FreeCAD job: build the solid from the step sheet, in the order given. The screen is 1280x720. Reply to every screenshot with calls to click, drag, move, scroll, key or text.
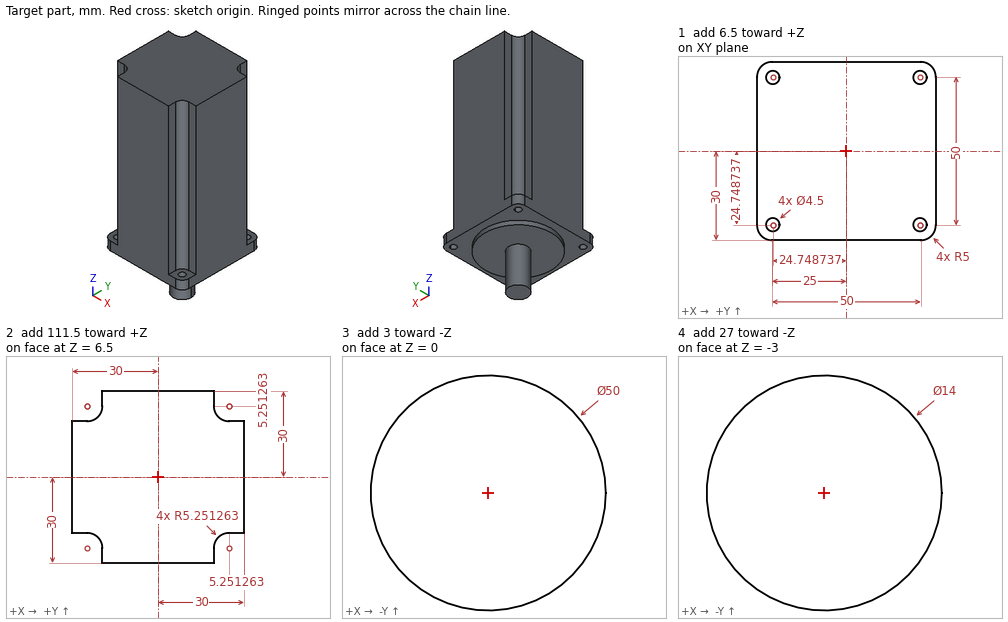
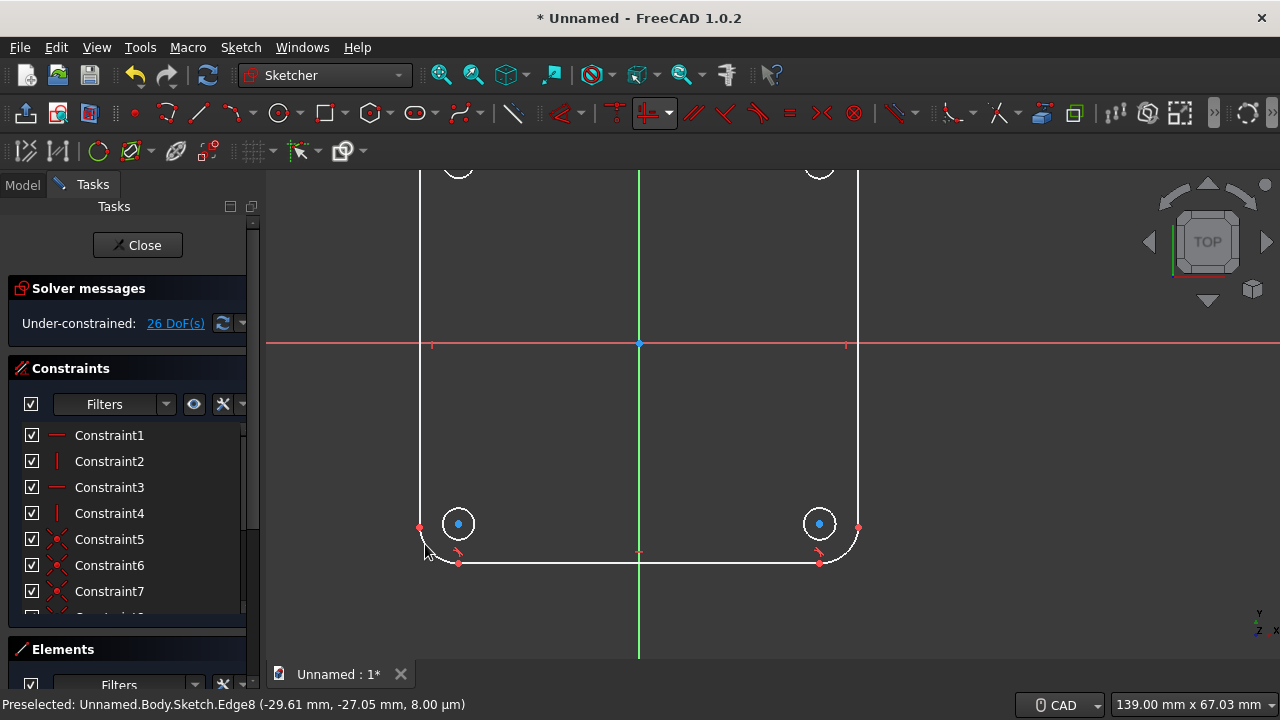
click(858, 418)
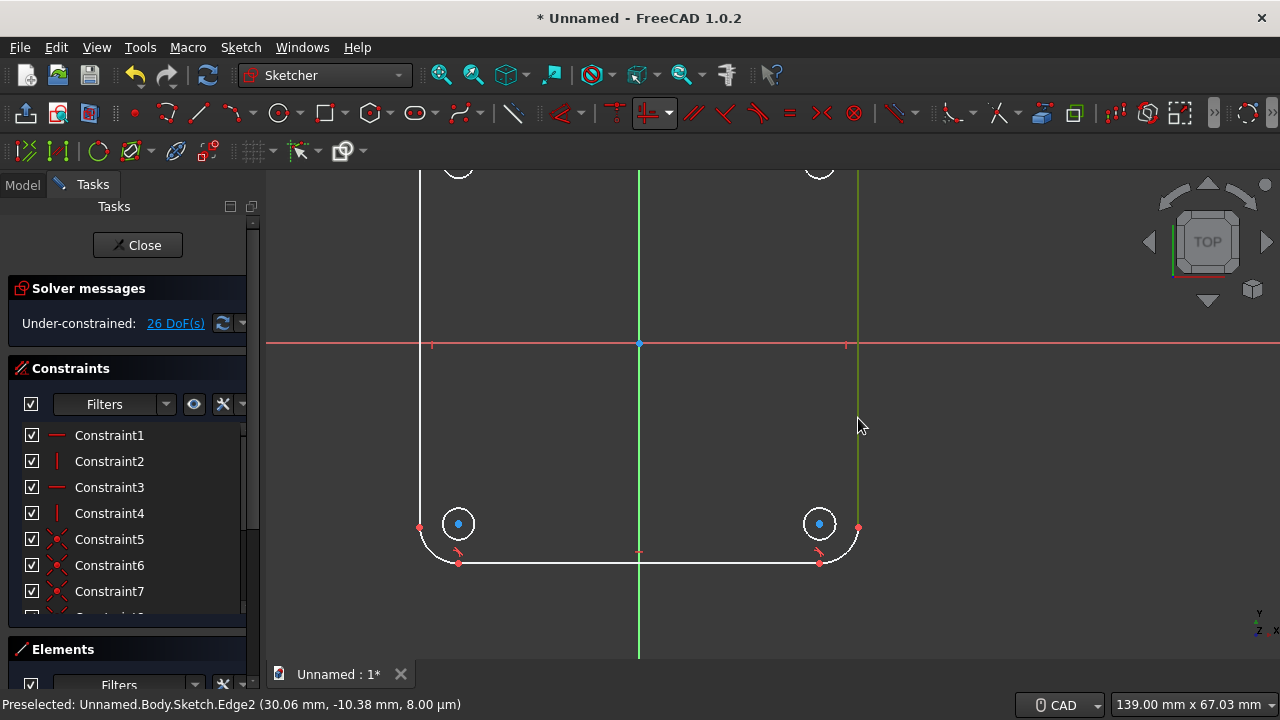
click(837, 560)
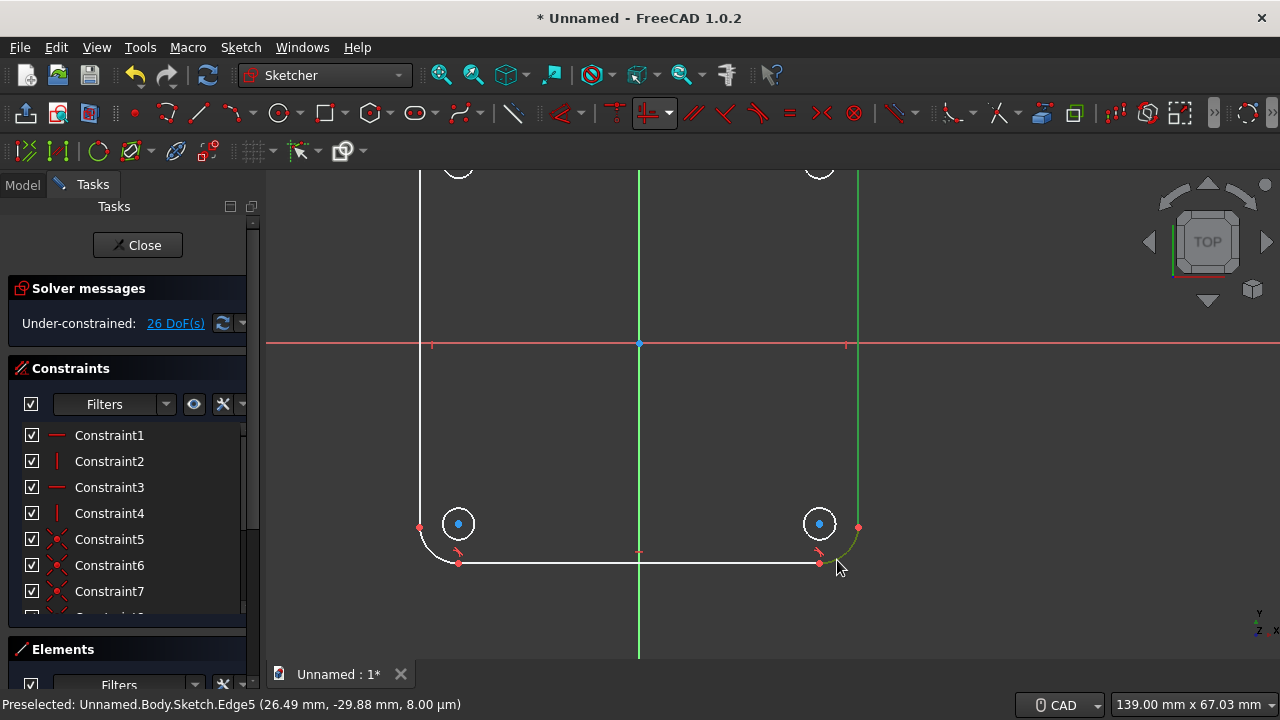
key(t)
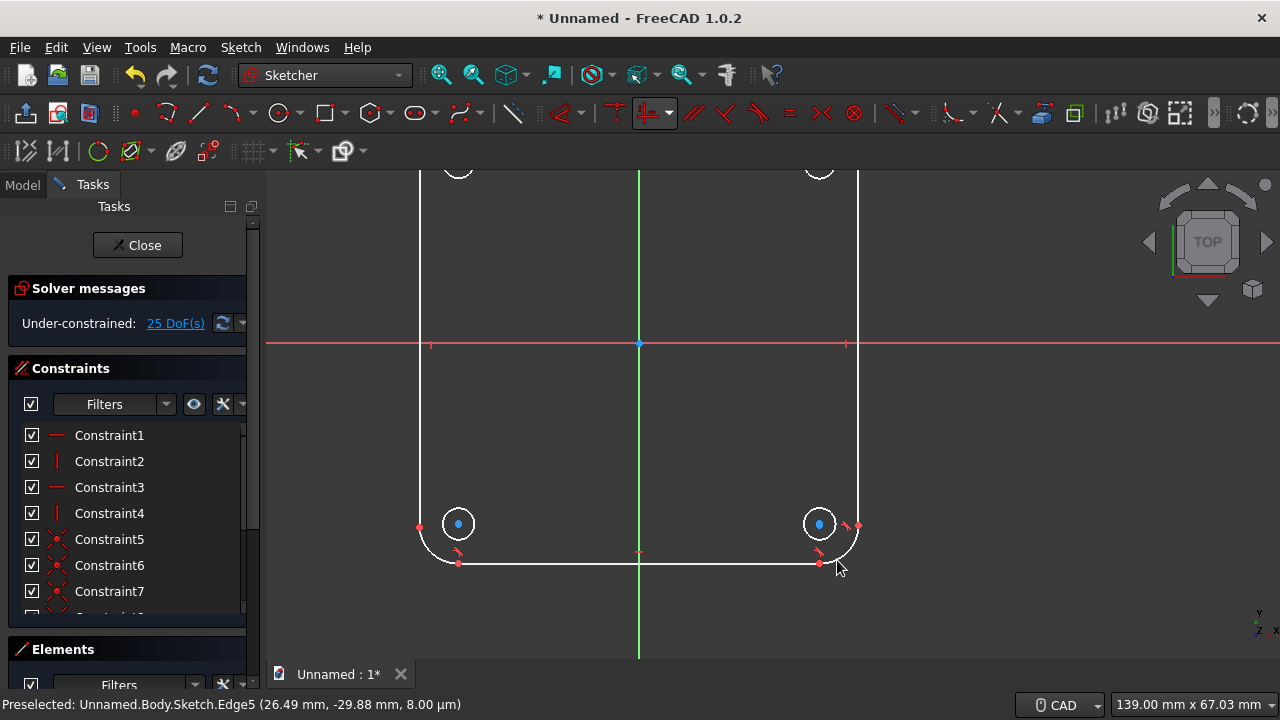
click(858, 416)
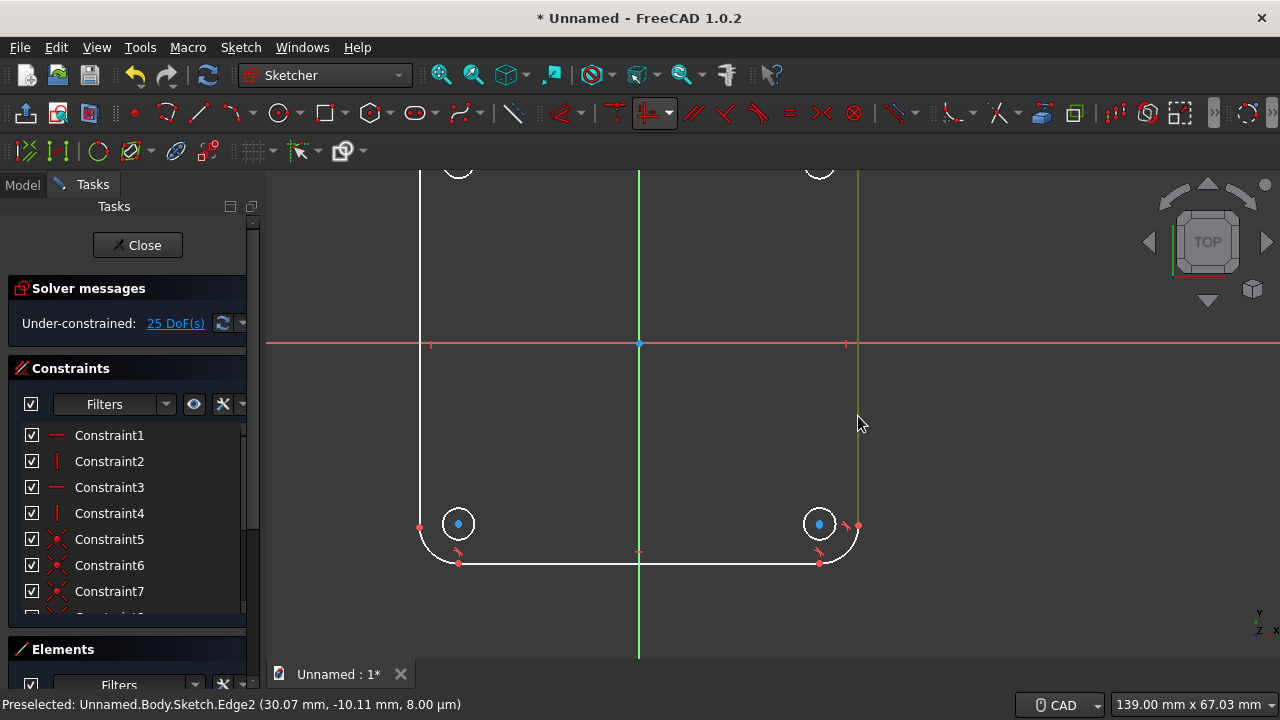
scroll(837, 559, down, 2)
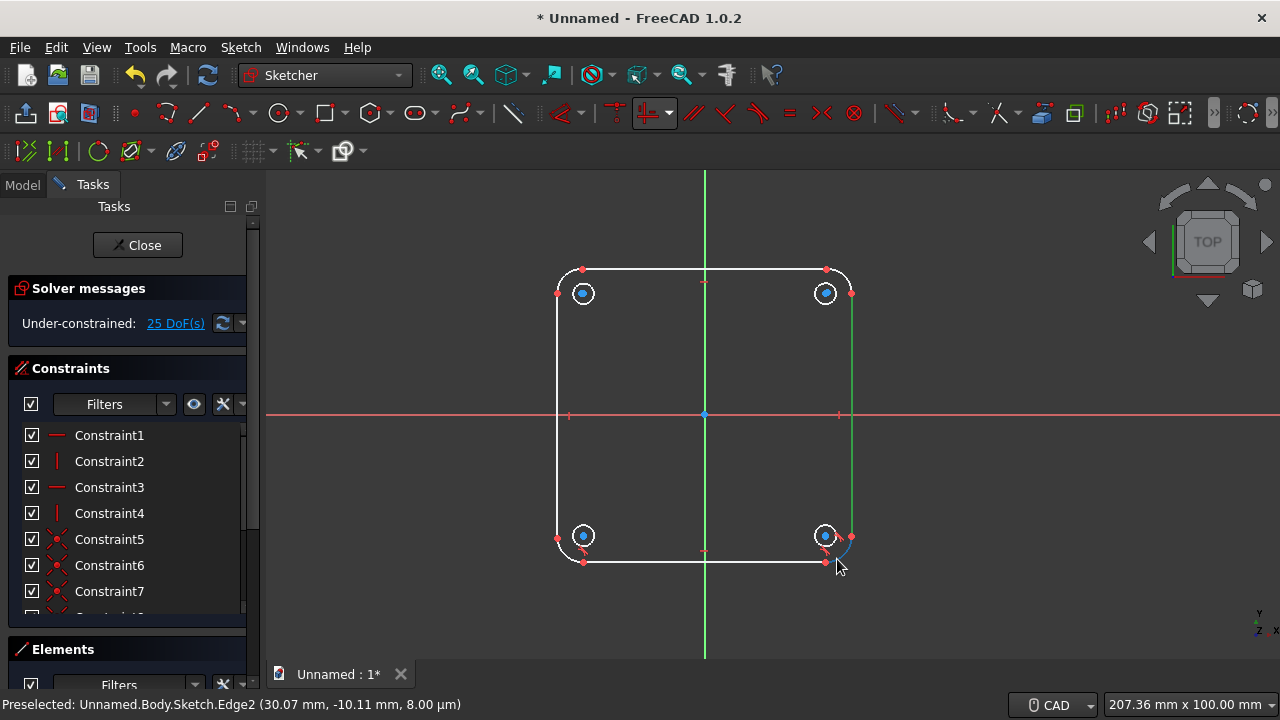
click(849, 282)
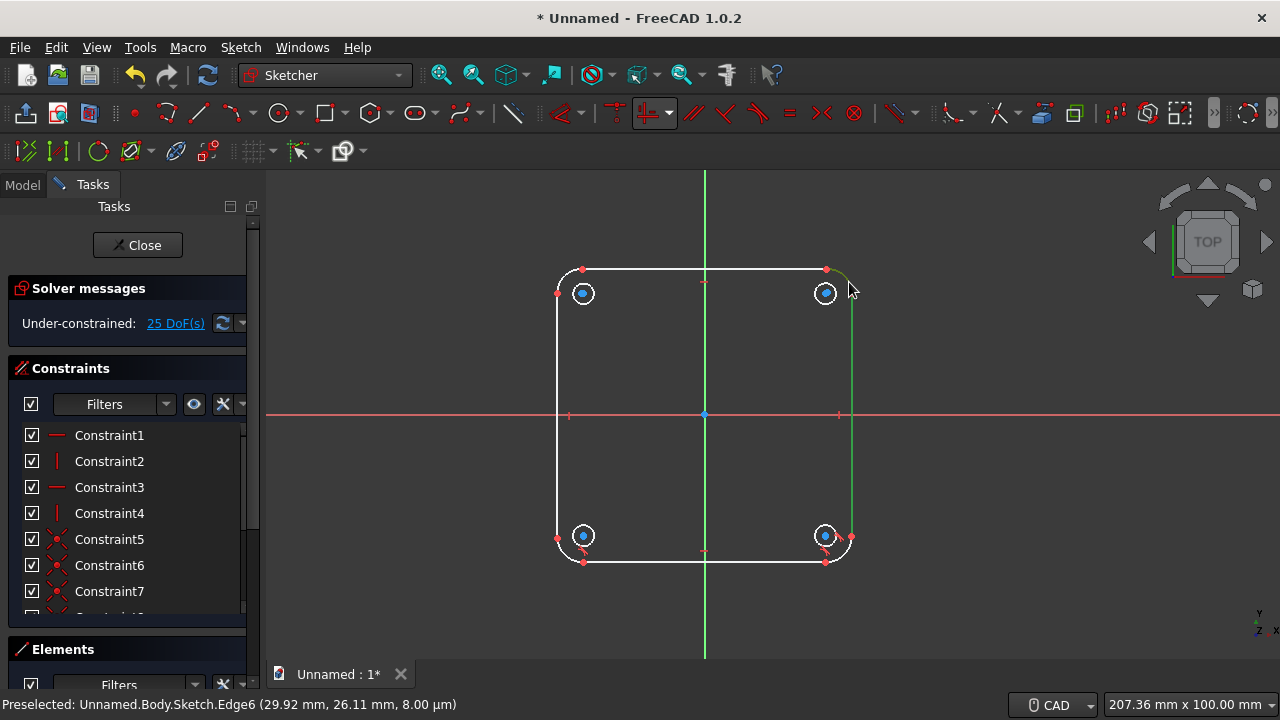
key(t)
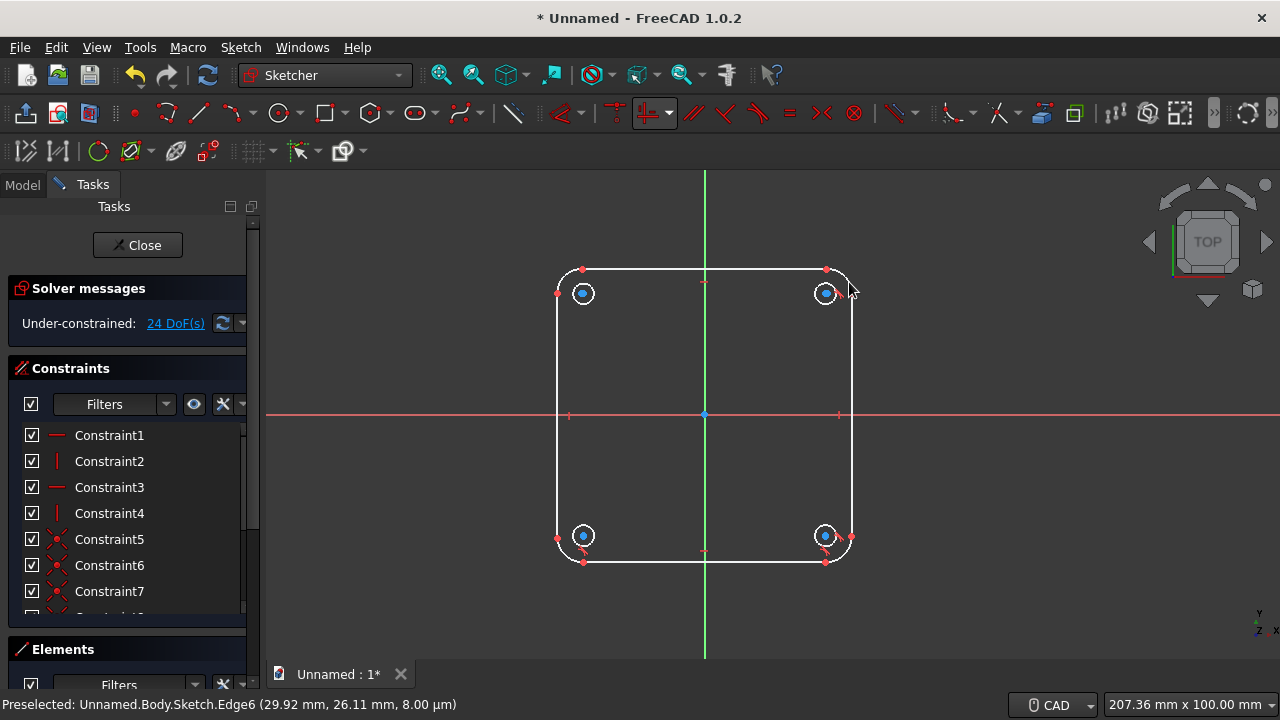
click(753, 269)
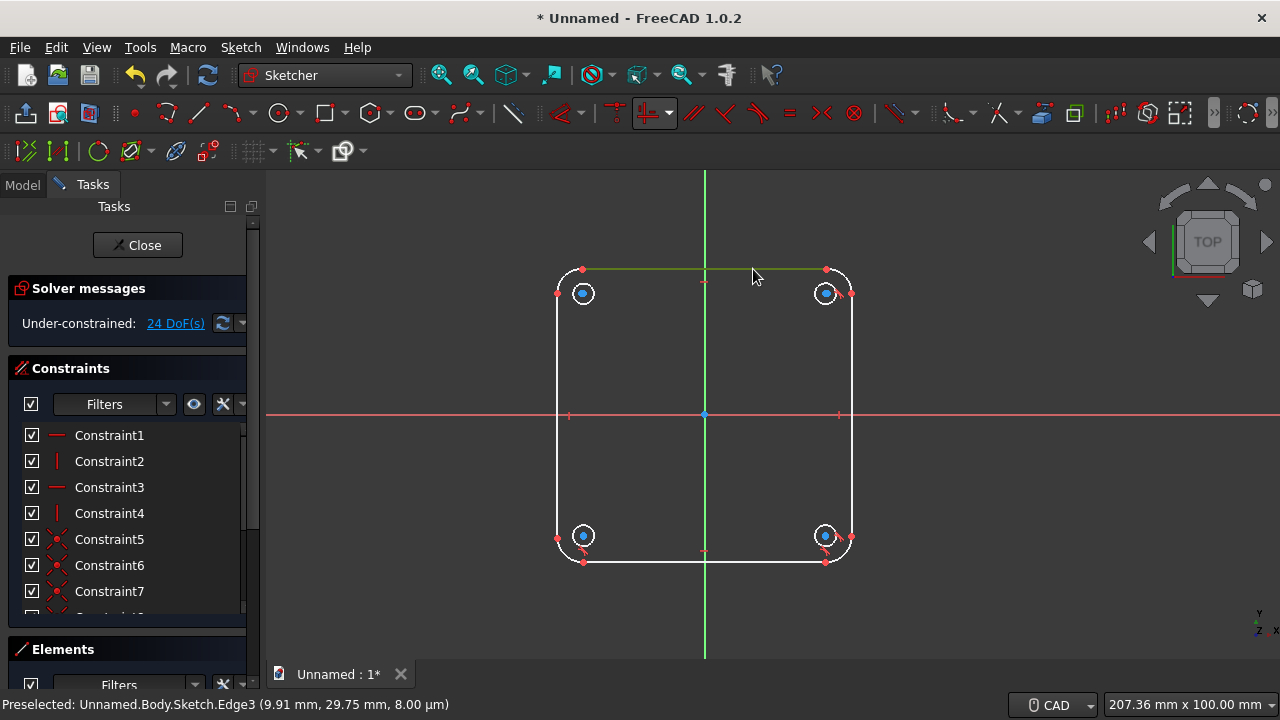
click(849, 282)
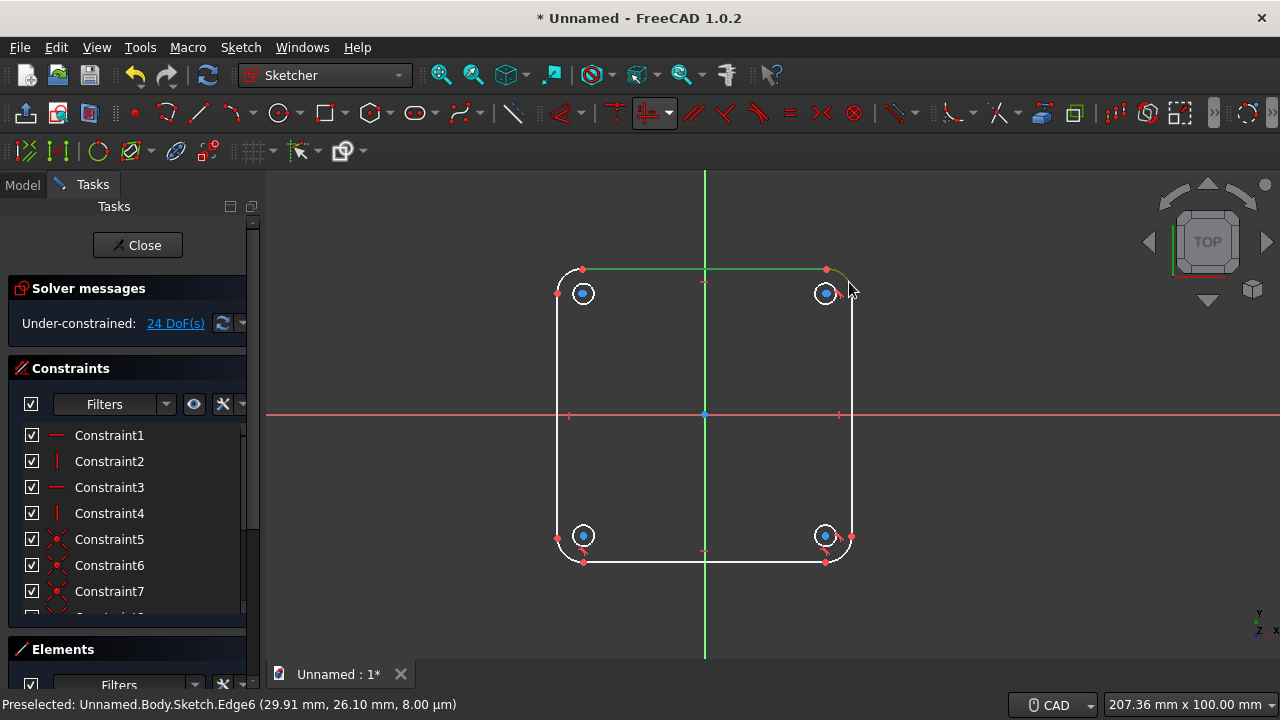
key(t)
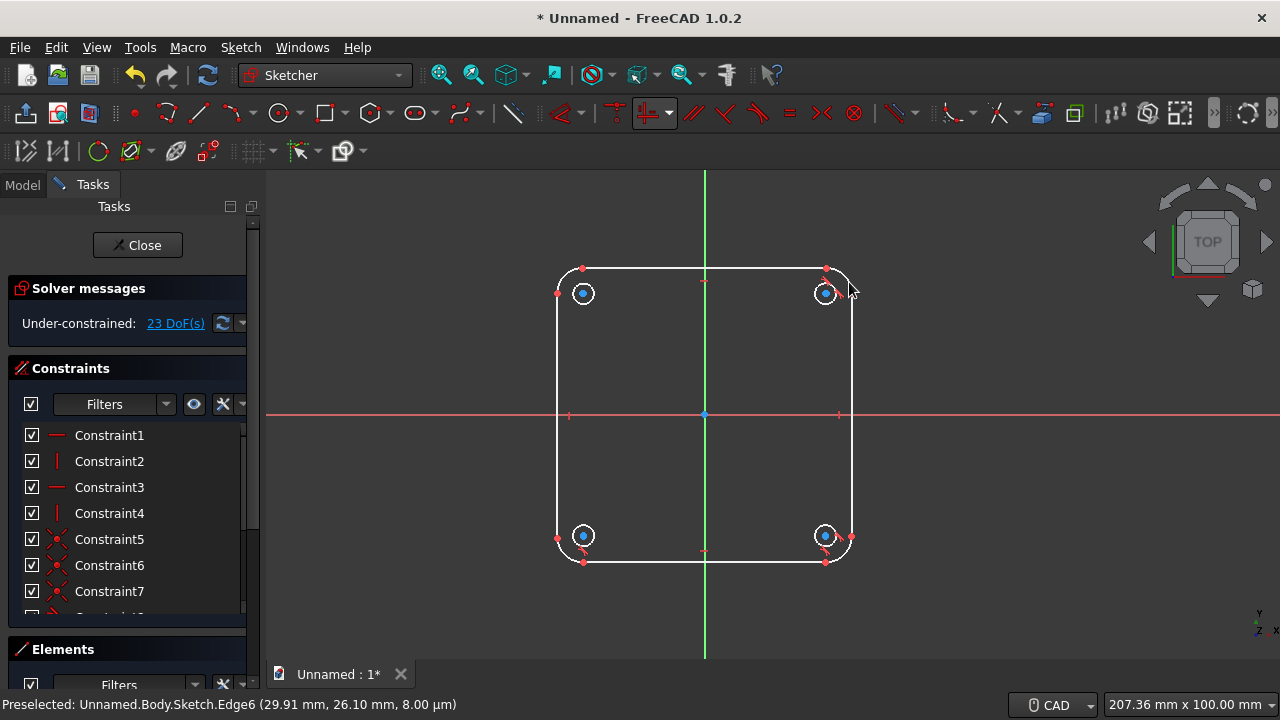
click(753, 268)